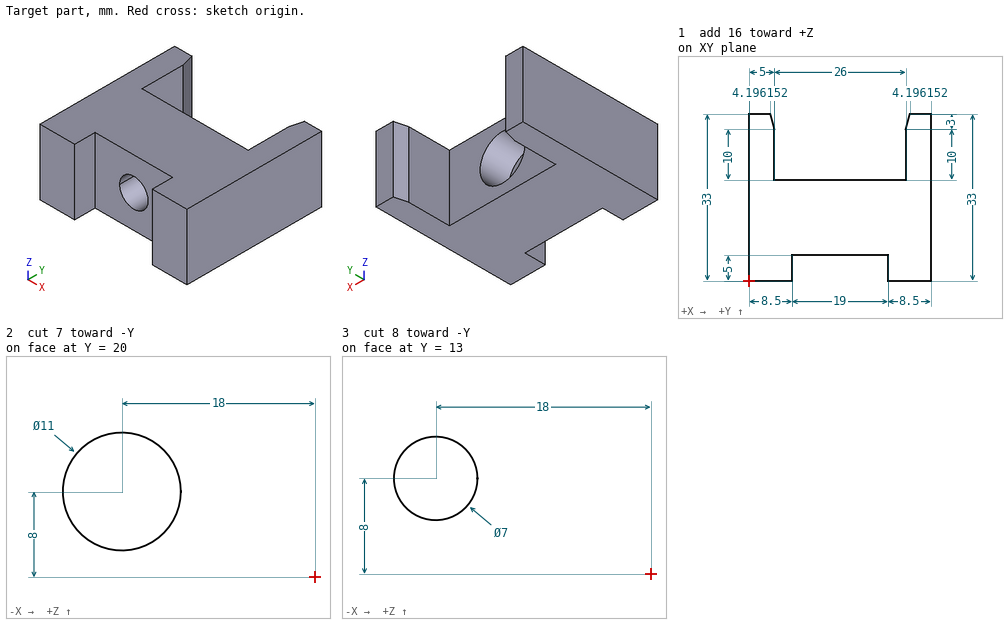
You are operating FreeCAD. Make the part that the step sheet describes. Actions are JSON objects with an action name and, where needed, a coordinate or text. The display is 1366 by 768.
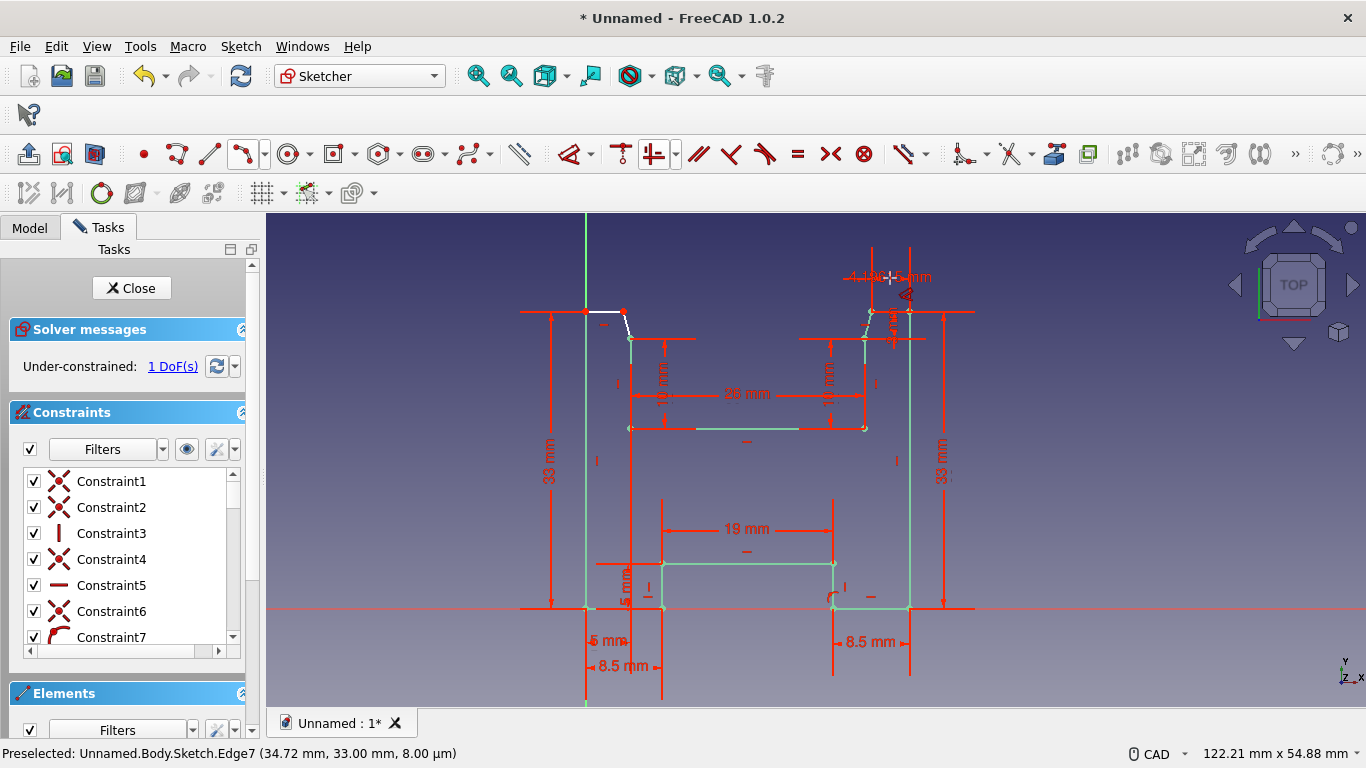
{"action": "left_click", "coordinate": [612, 312]}
{"action": "left_click", "coordinate": [604, 278]}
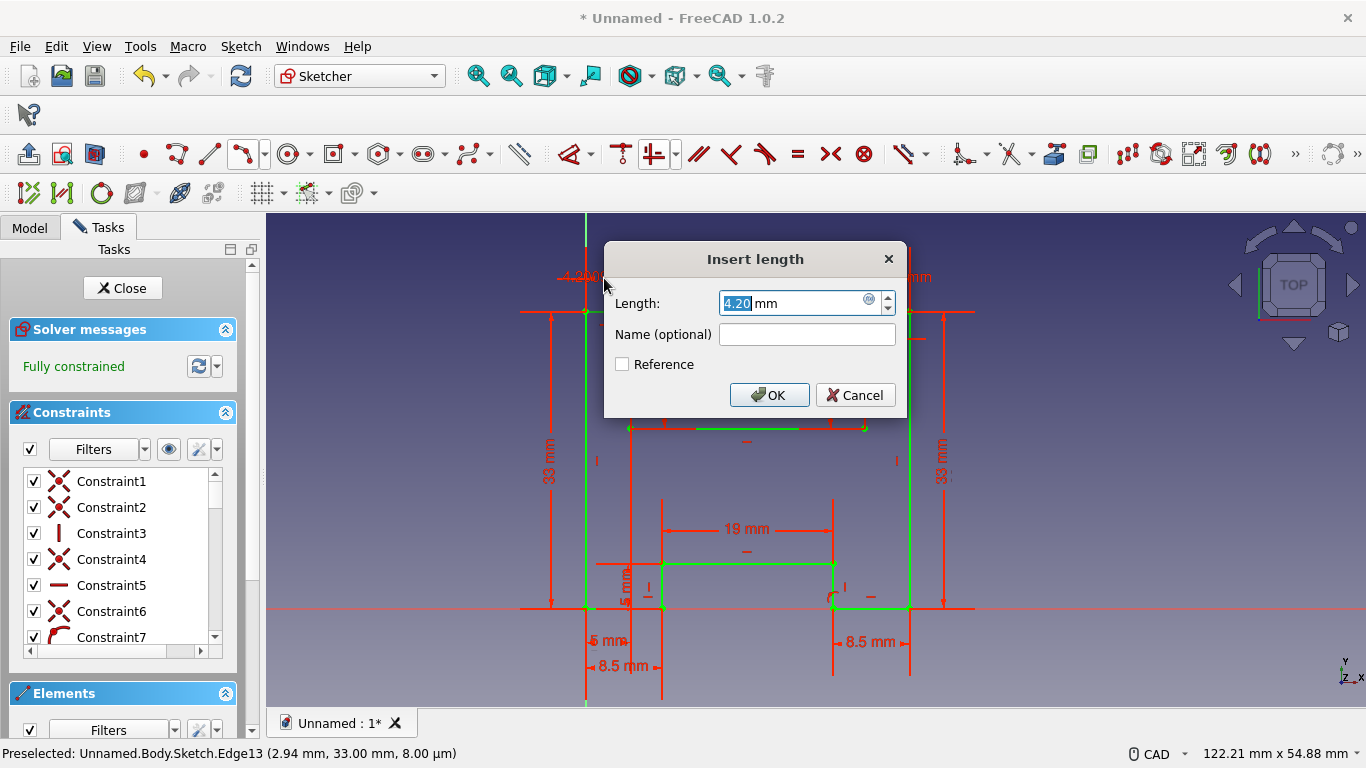
{"action": "type", "text": "4.196152"}
{"action": "key", "text": "Return"}
{"action": "key", "text": "Escape"}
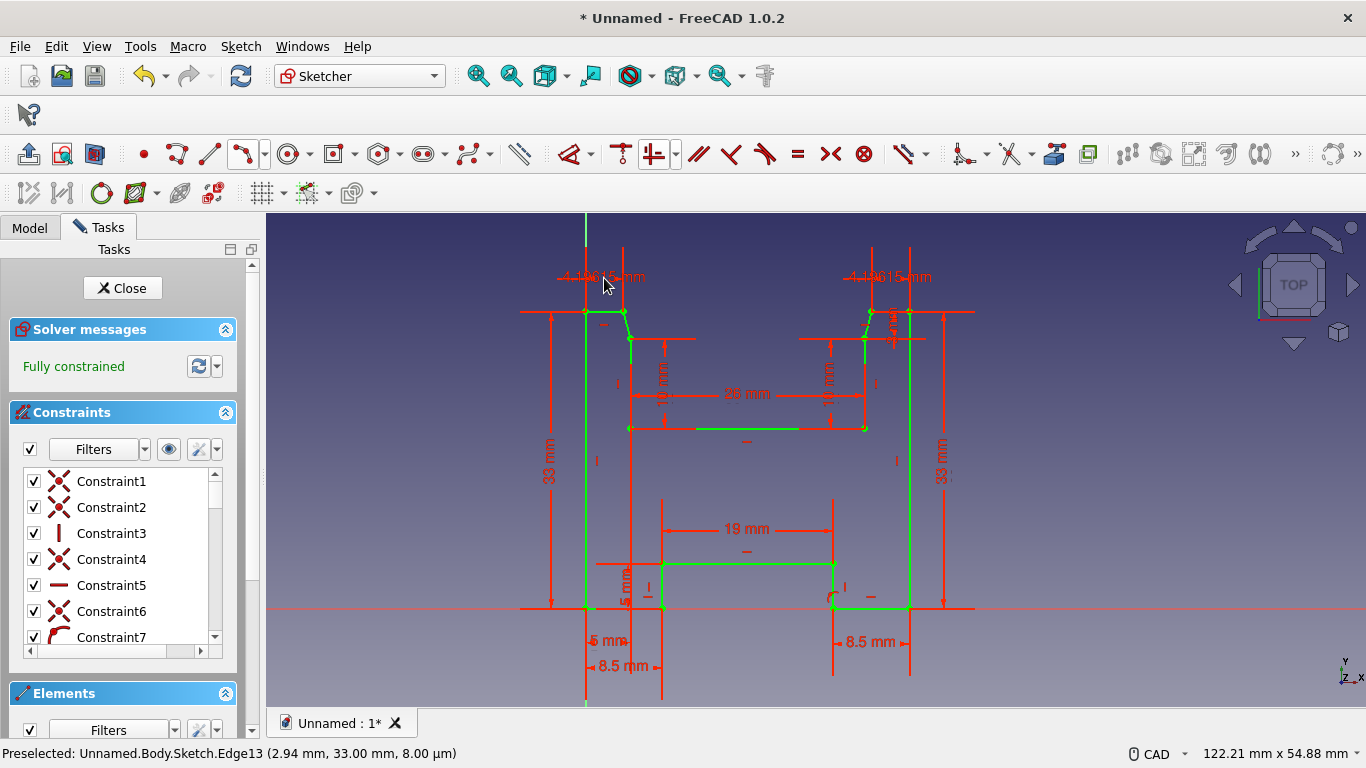
{"action": "left_click", "coordinate": [123, 288]}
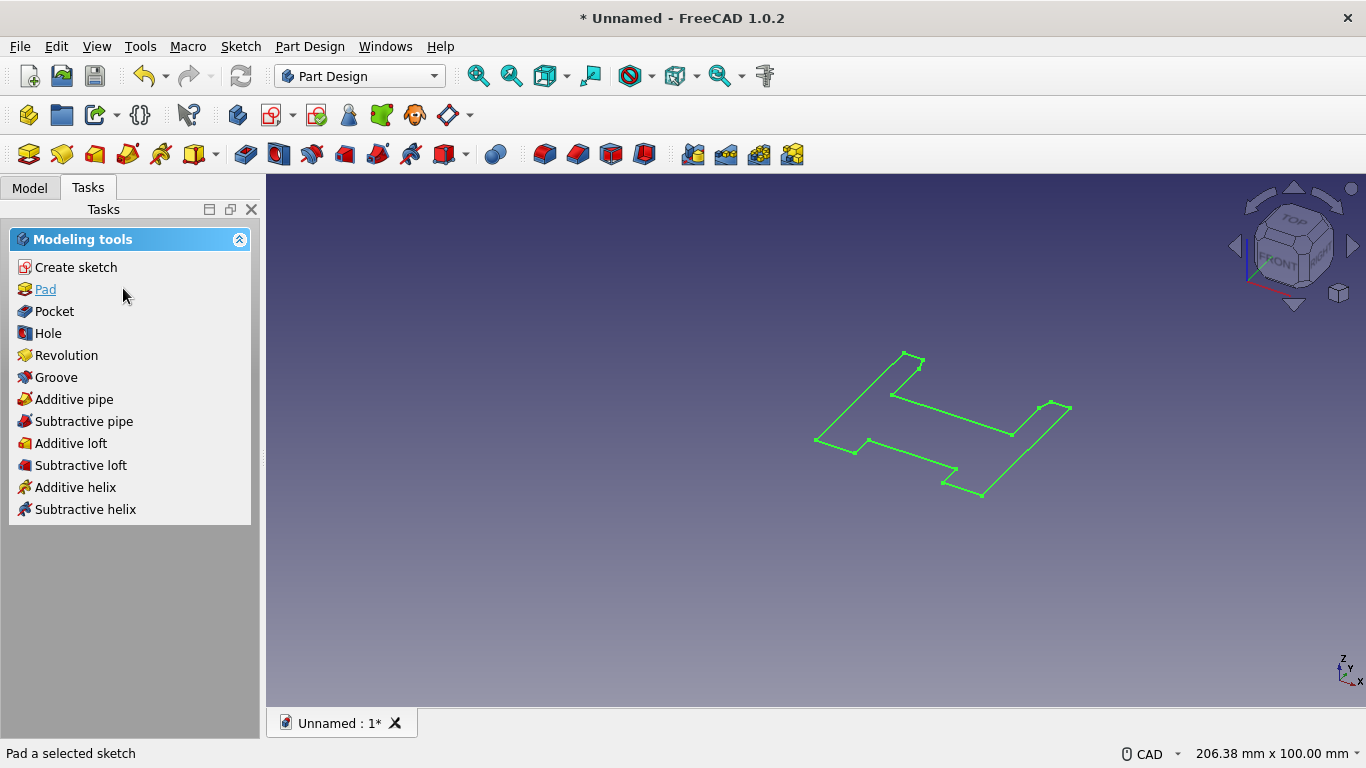
{"action": "left_click", "coordinate": [29, 154]}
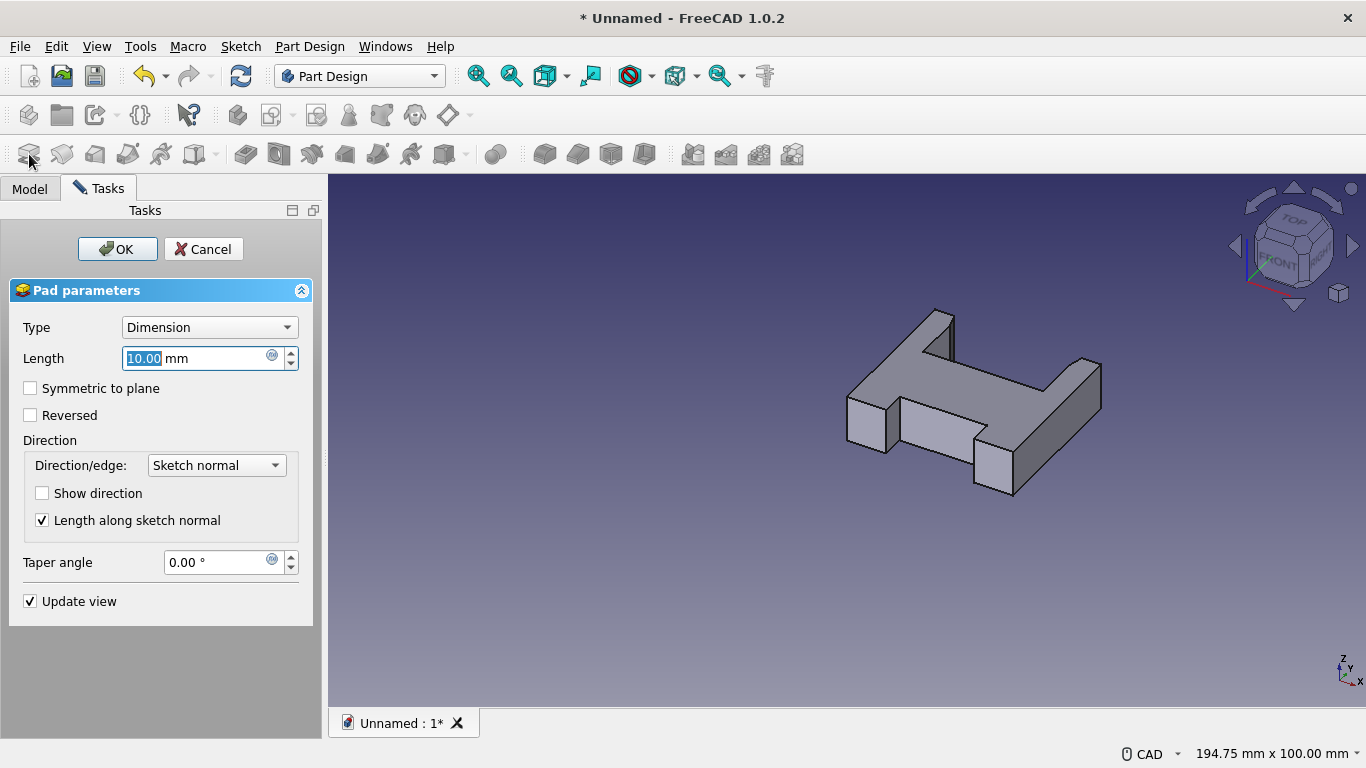
{"action": "type", "text": "16"}
{"action": "key", "text": "Tab"}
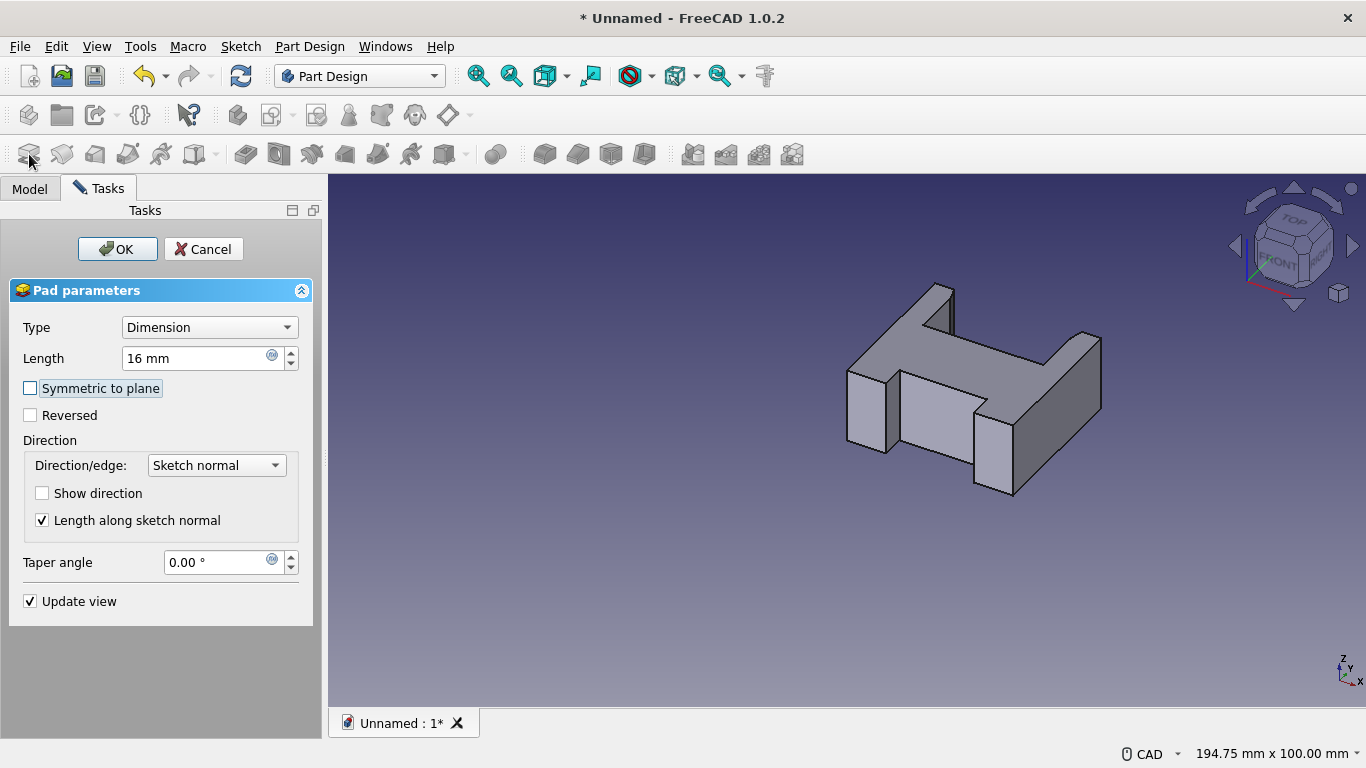
{"action": "left_click", "coordinate": [118, 249]}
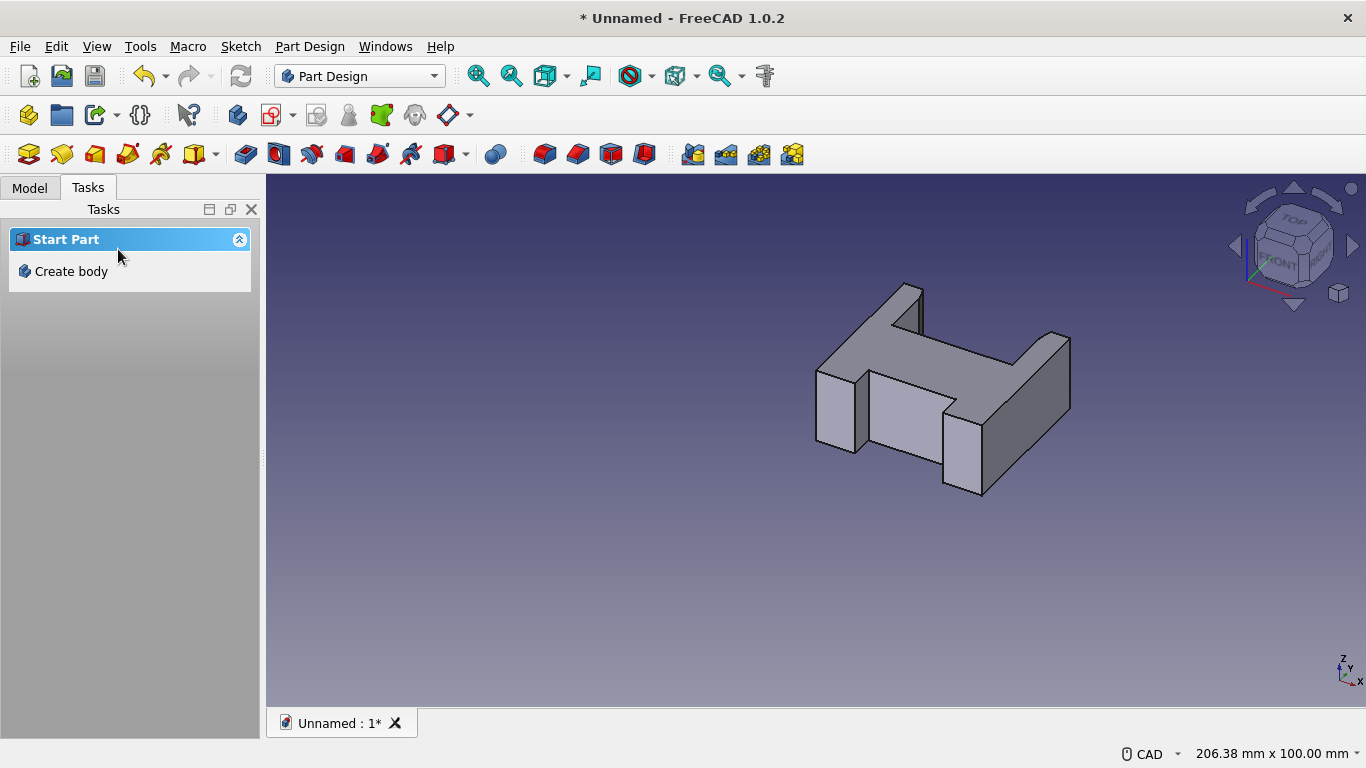
{"action": "left_click", "coordinate": [479, 76]}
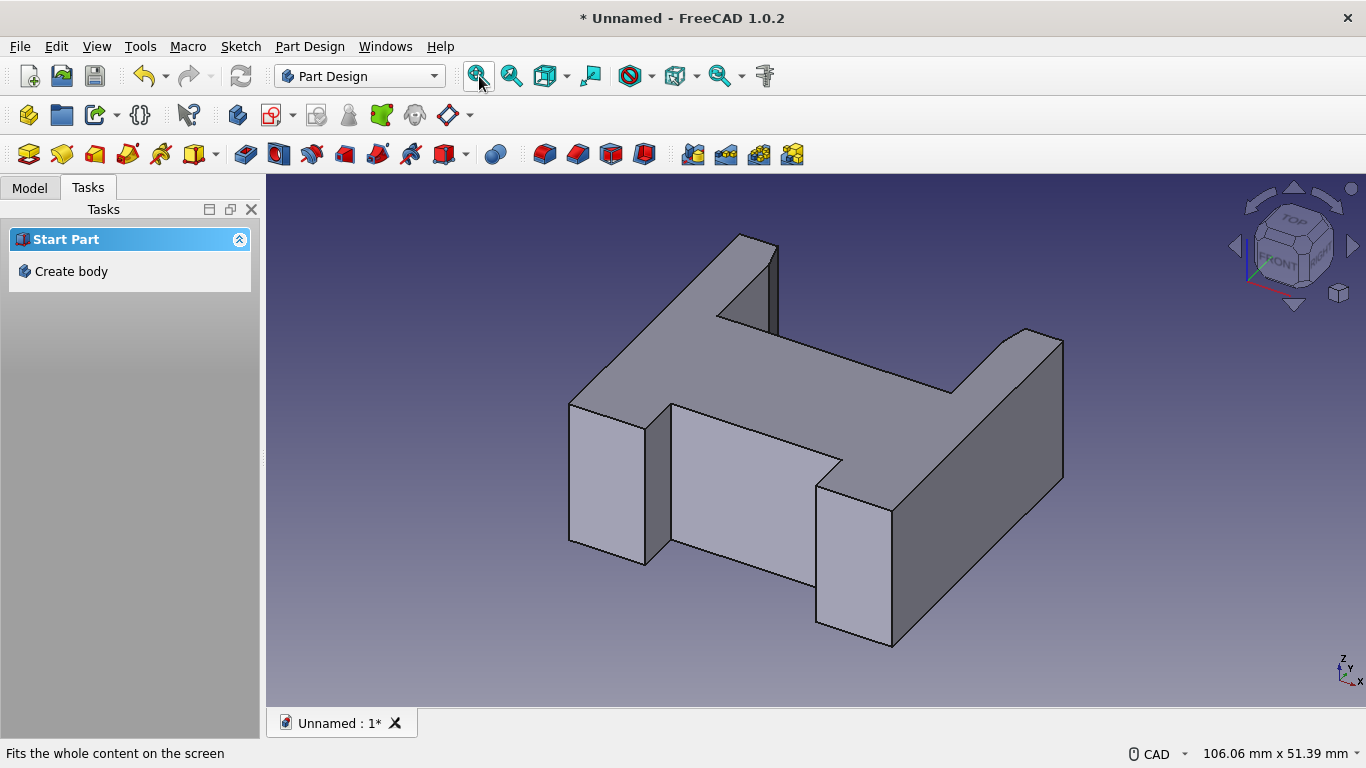
{"action": "key", "text": "4"}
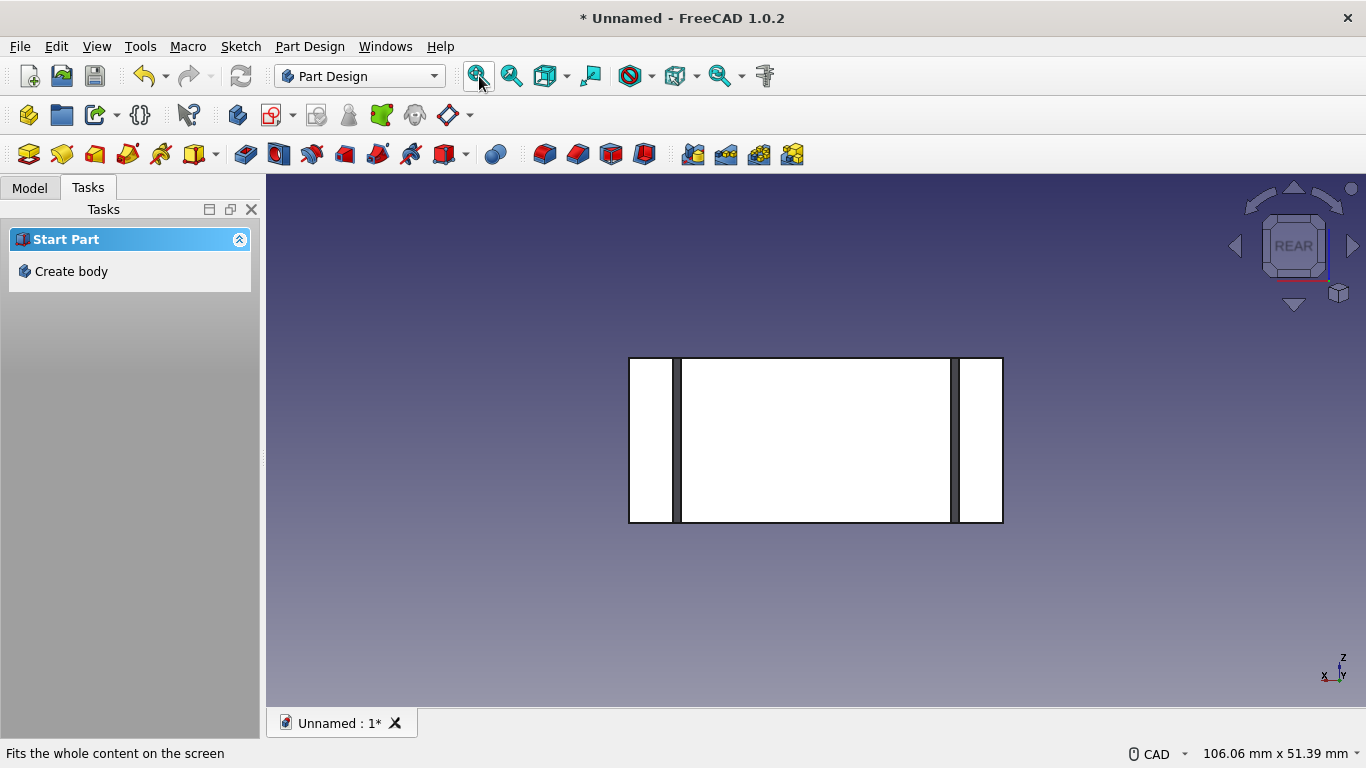
{"action": "left_click", "coordinate": [479, 76]}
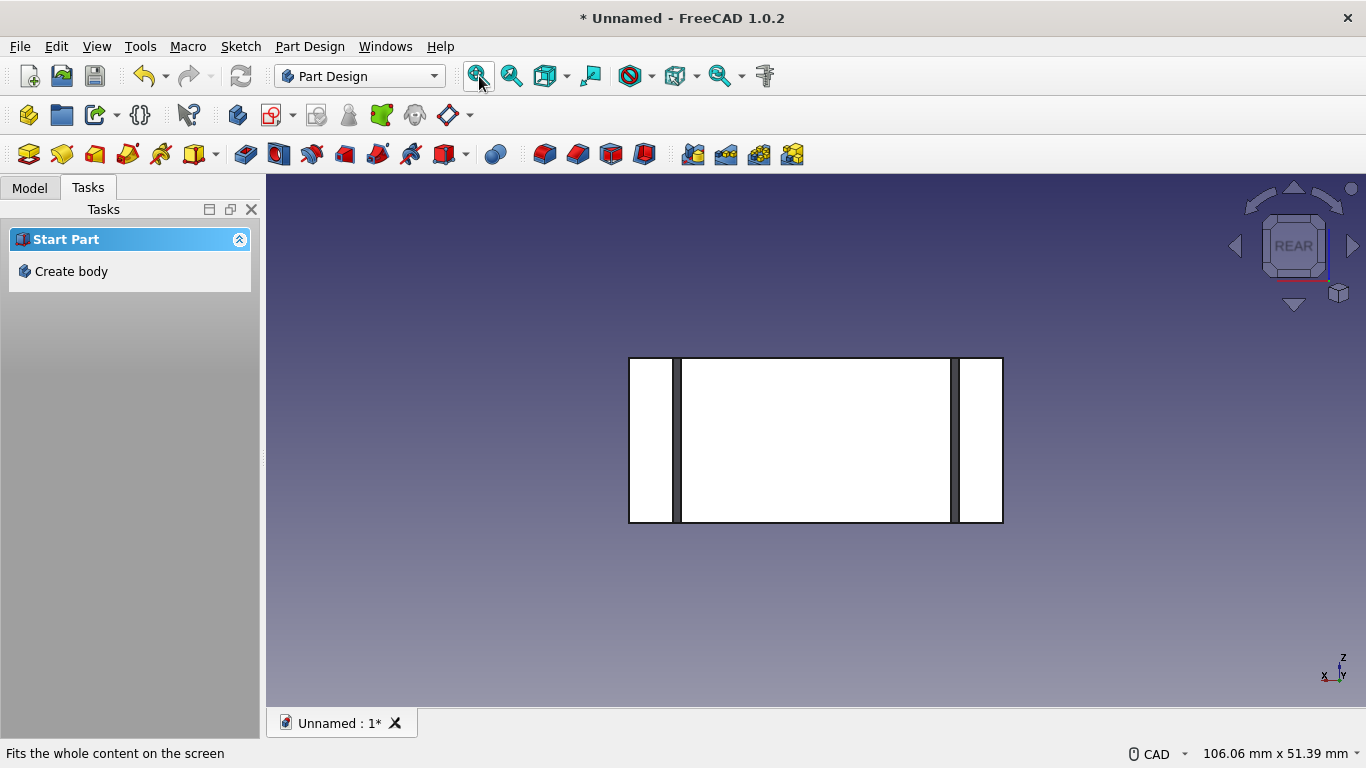
{"action": "left_click", "coordinate": [777, 440]}